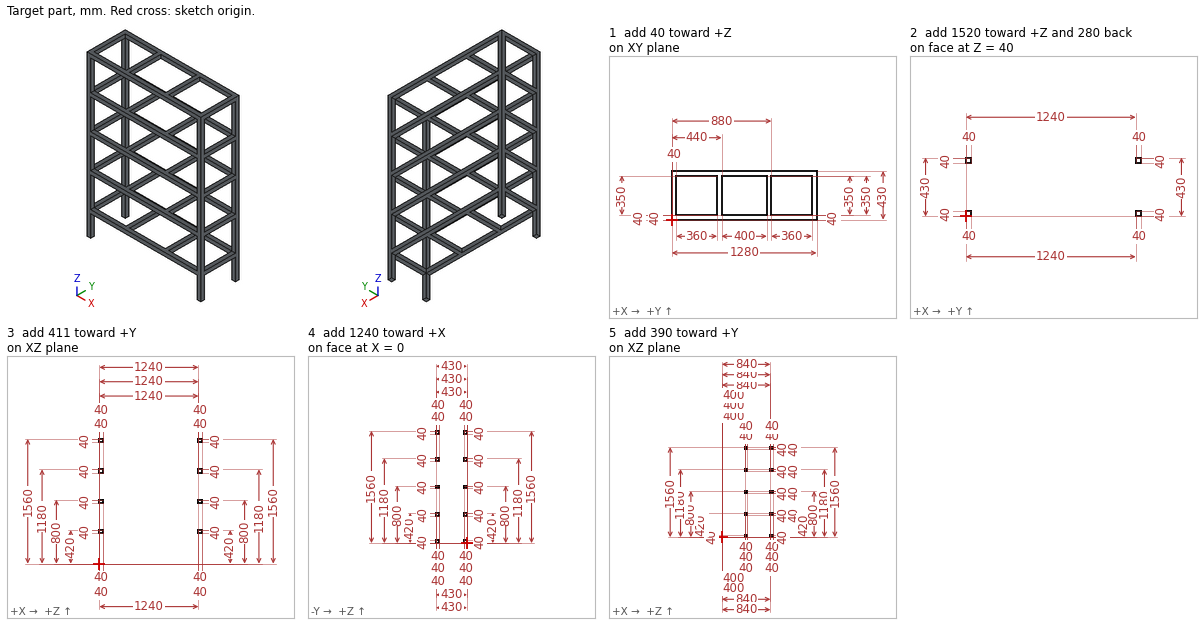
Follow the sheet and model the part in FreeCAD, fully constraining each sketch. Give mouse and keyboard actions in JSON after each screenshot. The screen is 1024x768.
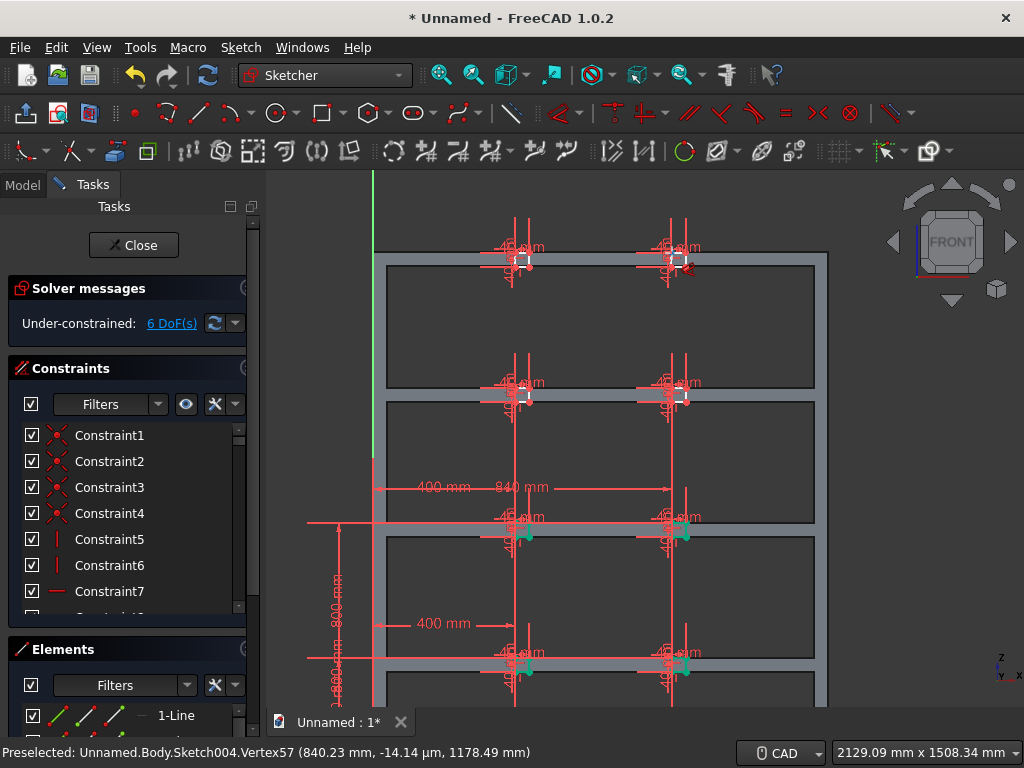
{"action": "left_click", "coordinate": [671, 253]}
{"action": "left_click", "coordinate": [522, 219]}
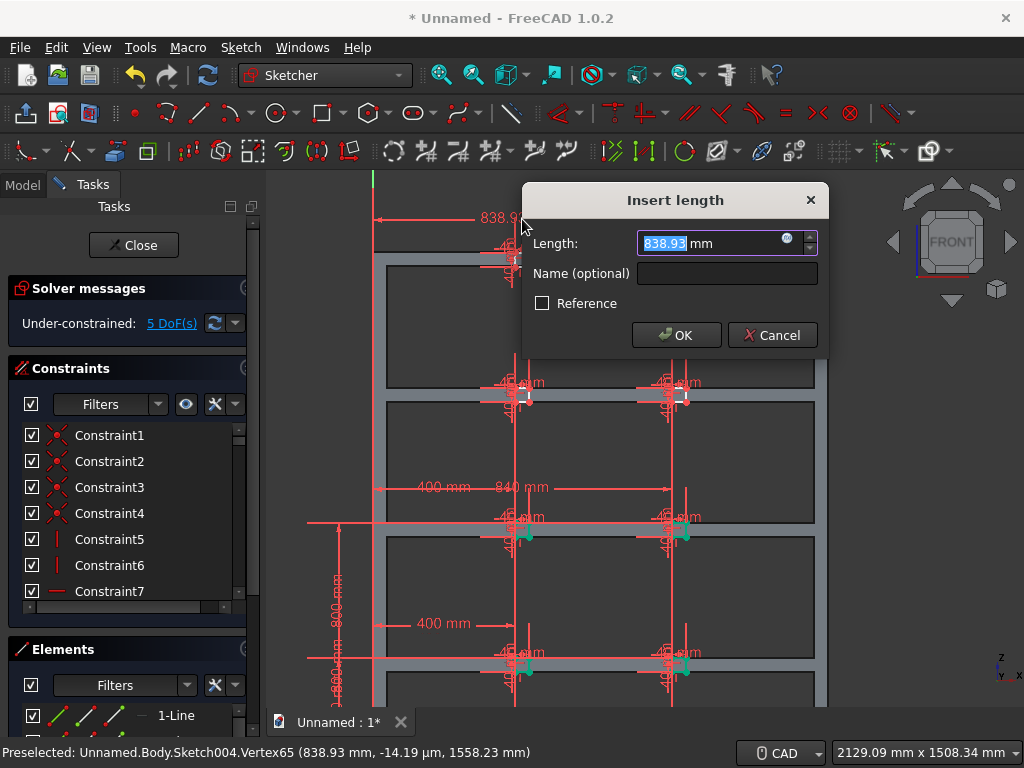
{"action": "type", "text": "840"}
{"action": "key", "text": "Return"}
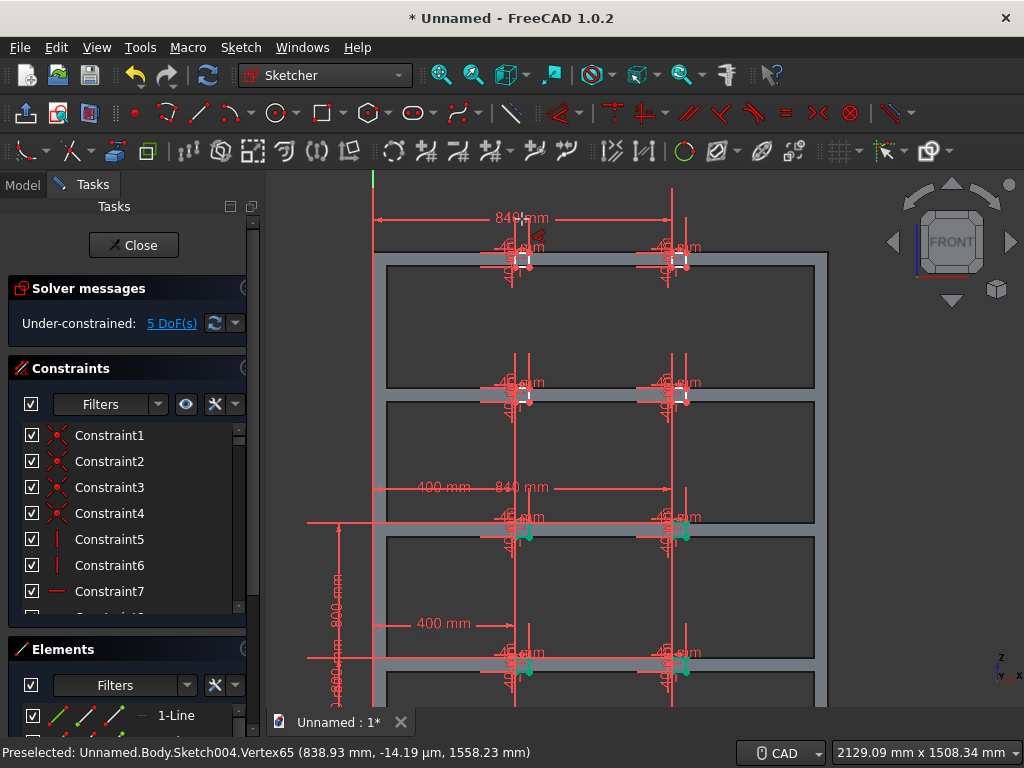
{"action": "left_click", "coordinate": [515, 253]}
{"action": "left_click", "coordinate": [444, 219]}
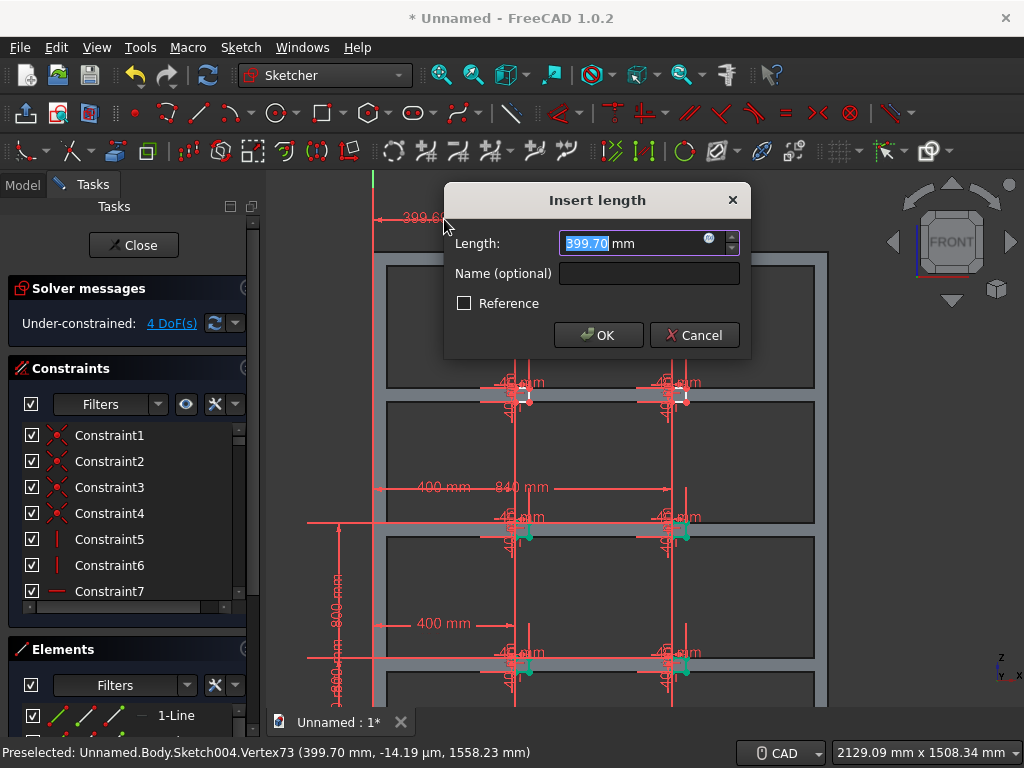
{"action": "type", "text": "400"}
{"action": "key", "text": "Return"}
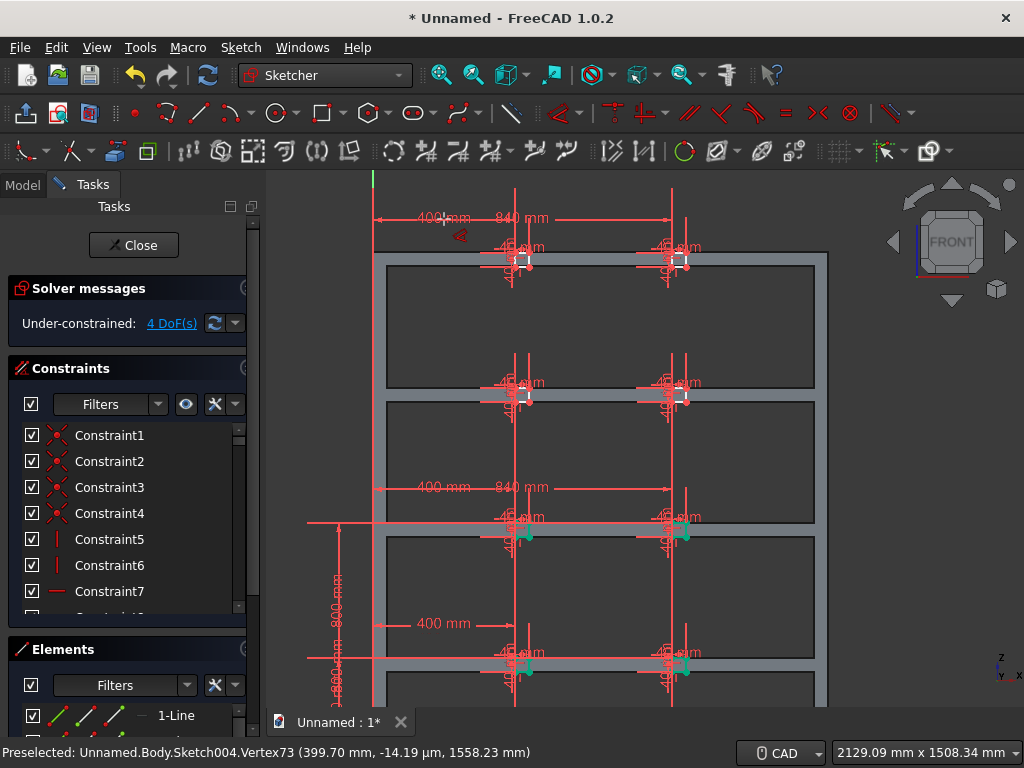
{"action": "left_click", "coordinate": [515, 388]}
{"action": "left_click", "coordinate": [339, 534]}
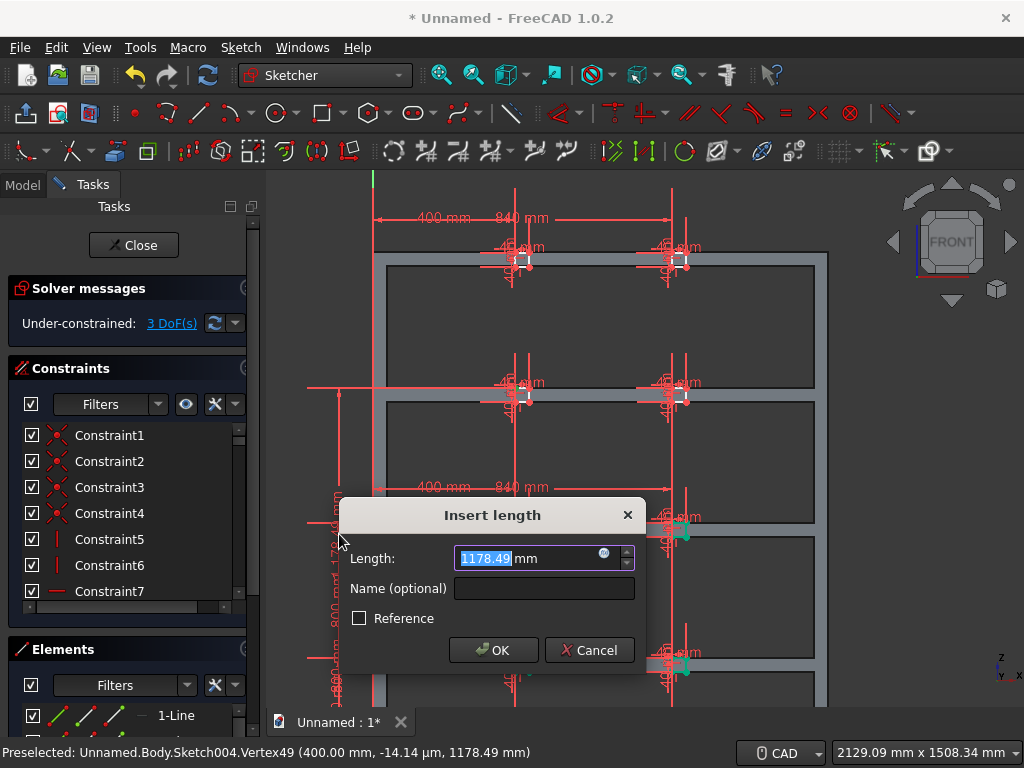
{"action": "type", "text": "1180"}
{"action": "key", "text": "Return"}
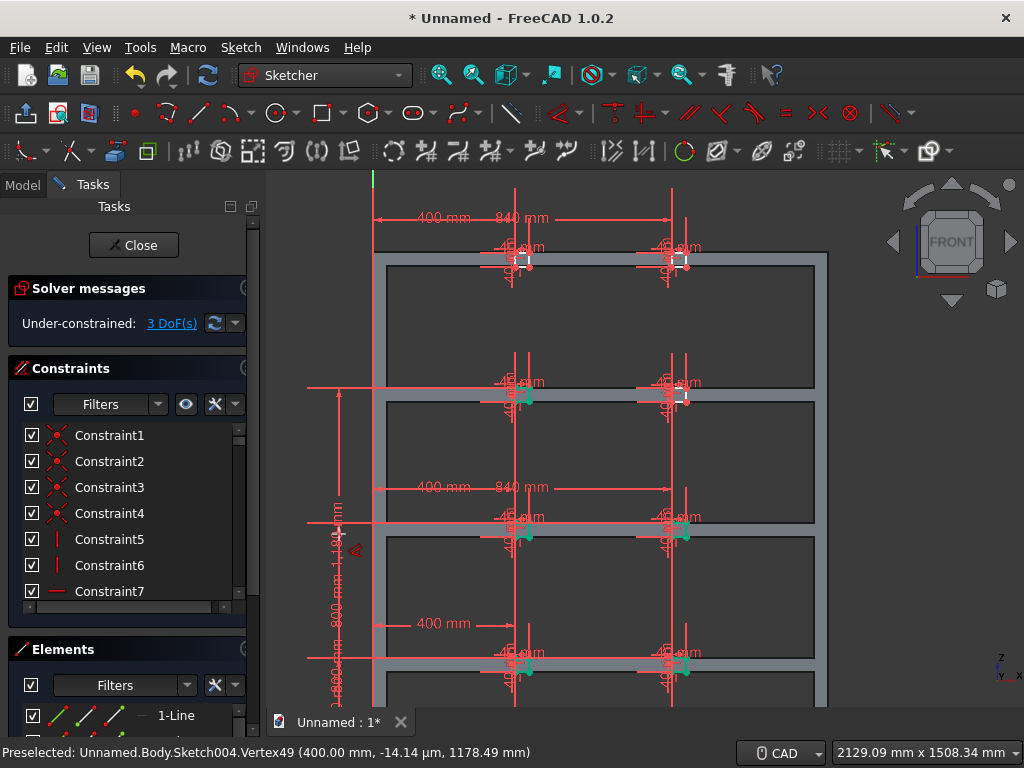
{"action": "left_click", "coordinate": [672, 388]}
{"action": "left_click", "coordinate": [339, 467]}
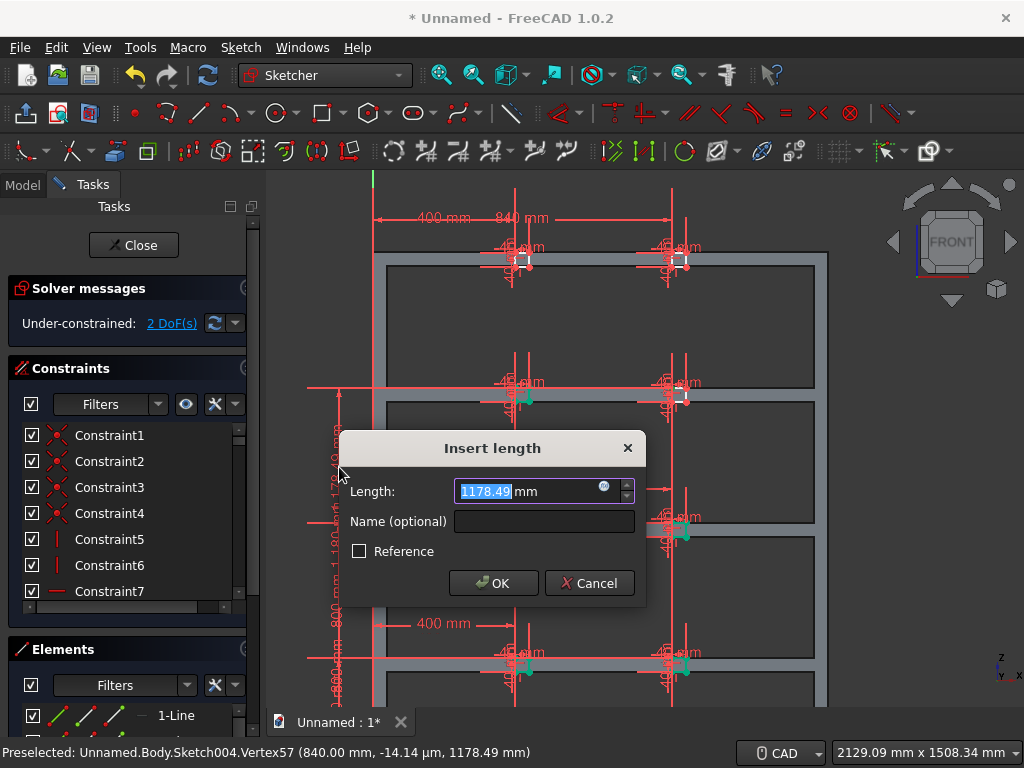
{"action": "type", "text": "1180"}
{"action": "key", "text": "Return"}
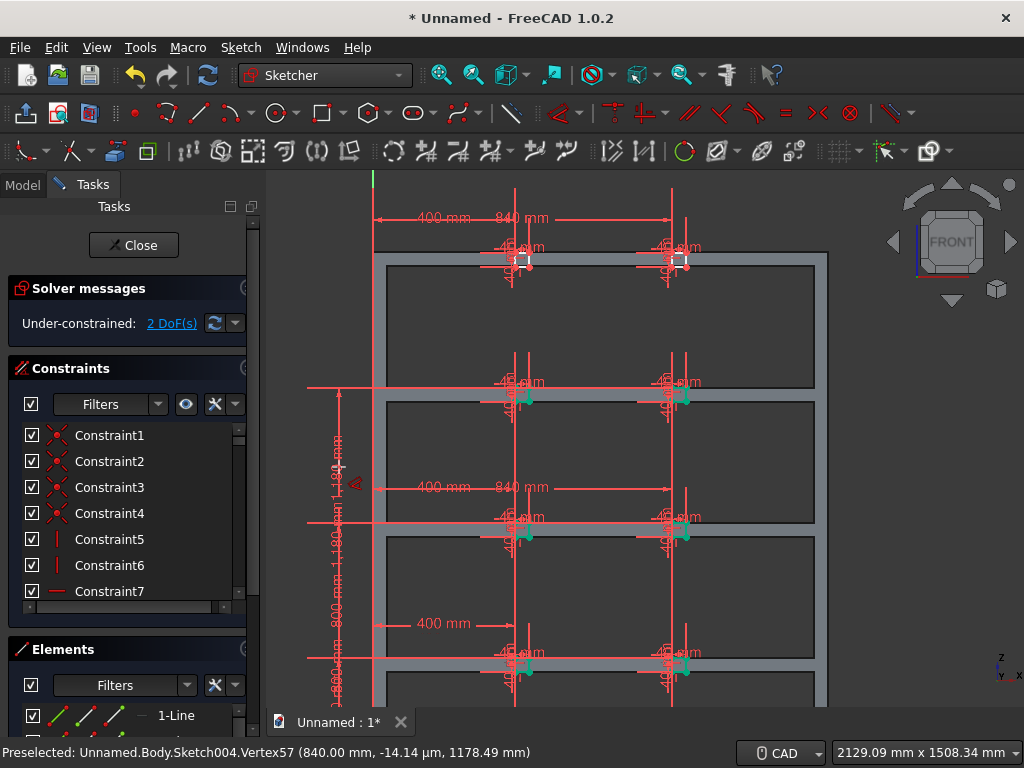
{"action": "left_click", "coordinate": [672, 253]}
{"action": "left_click", "coordinate": [339, 368]}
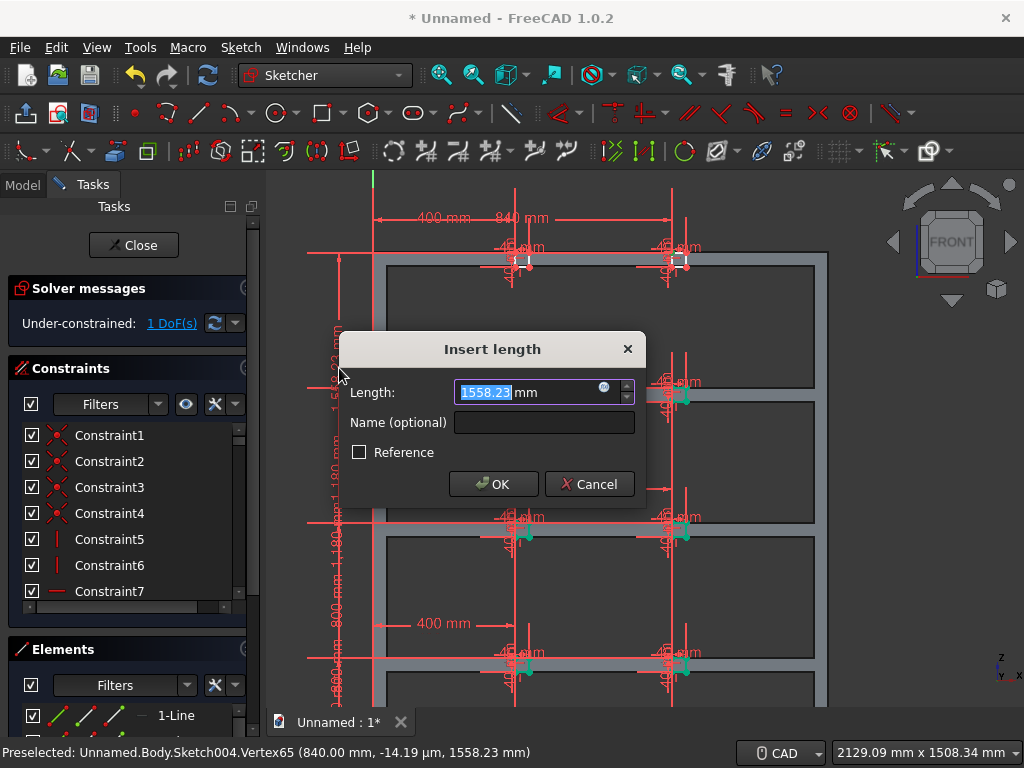
{"action": "type", "text": "1560"}
{"action": "key", "text": "Return"}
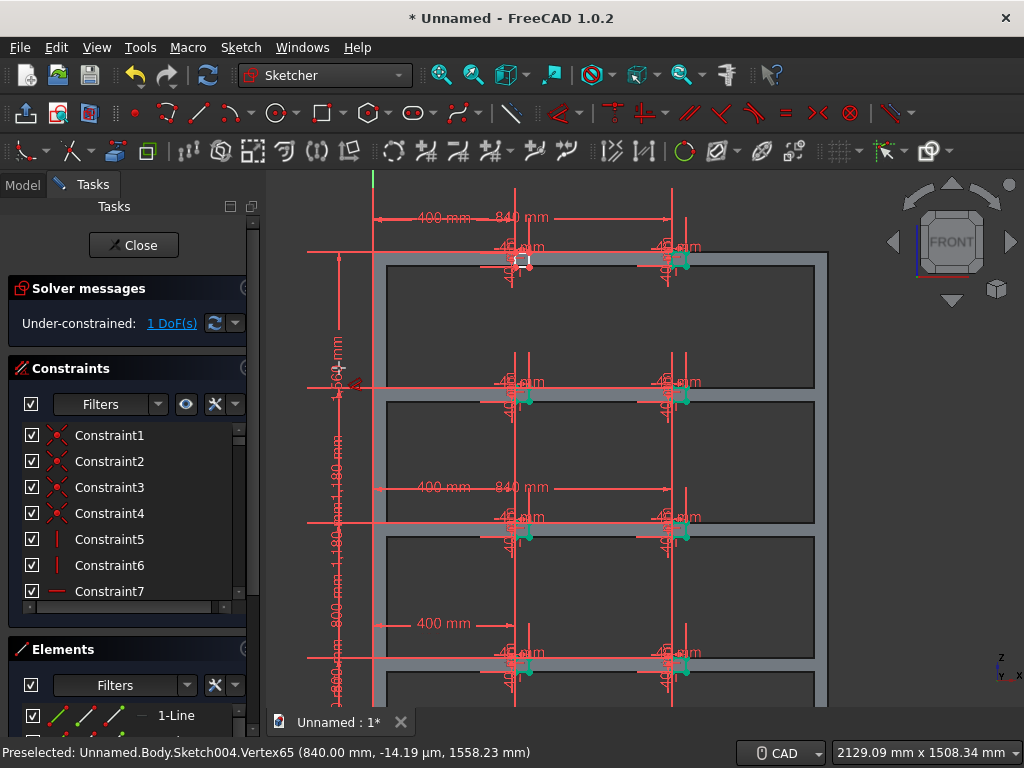
{"action": "left_click", "coordinate": [515, 253]}
{"action": "left_click", "coordinate": [339, 564]}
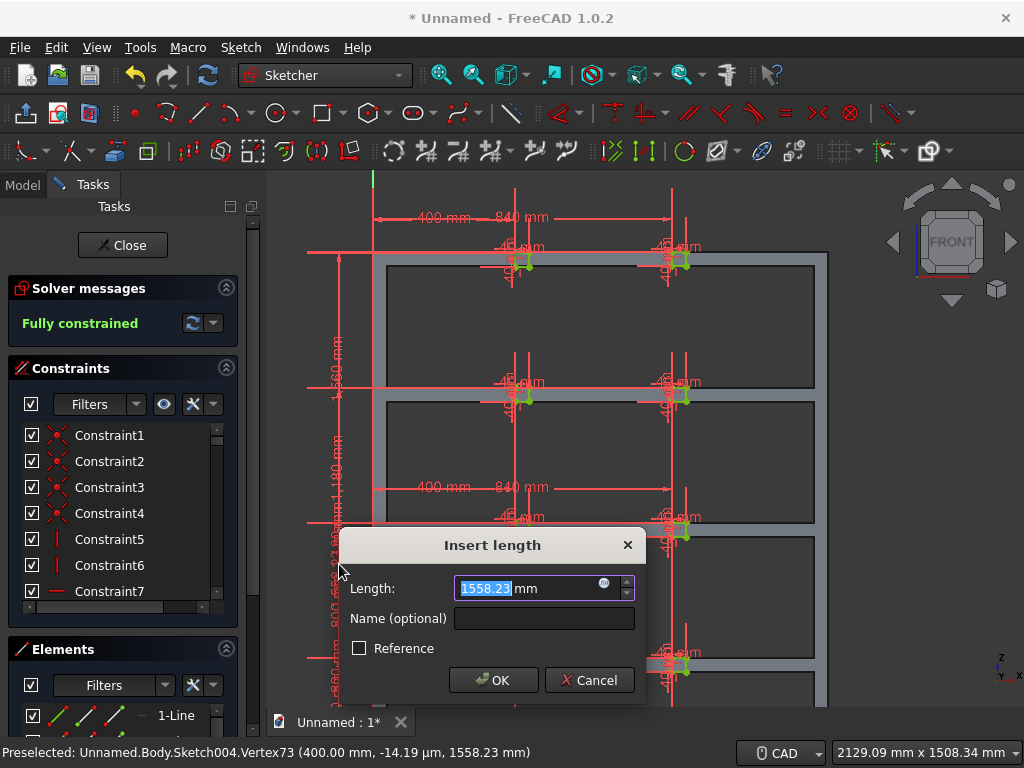
{"action": "type", "text": "1560"}
{"action": "key", "text": "Return"}
{"action": "key", "text": "Escape"}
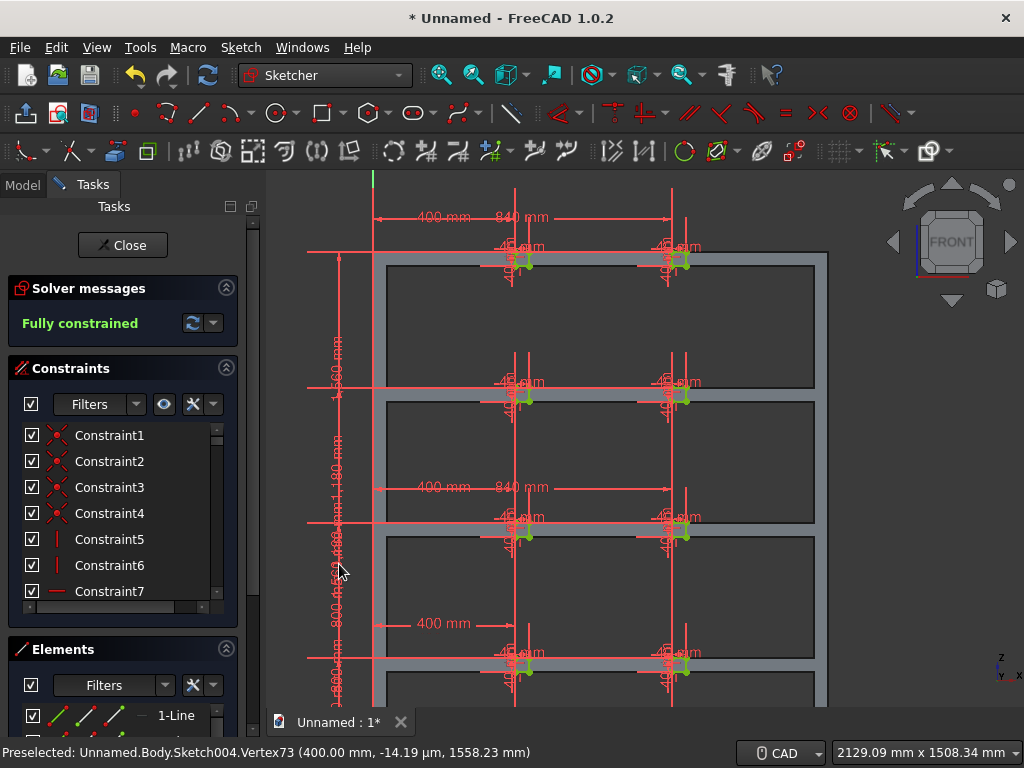
{"action": "left_click", "coordinate": [123, 245]}